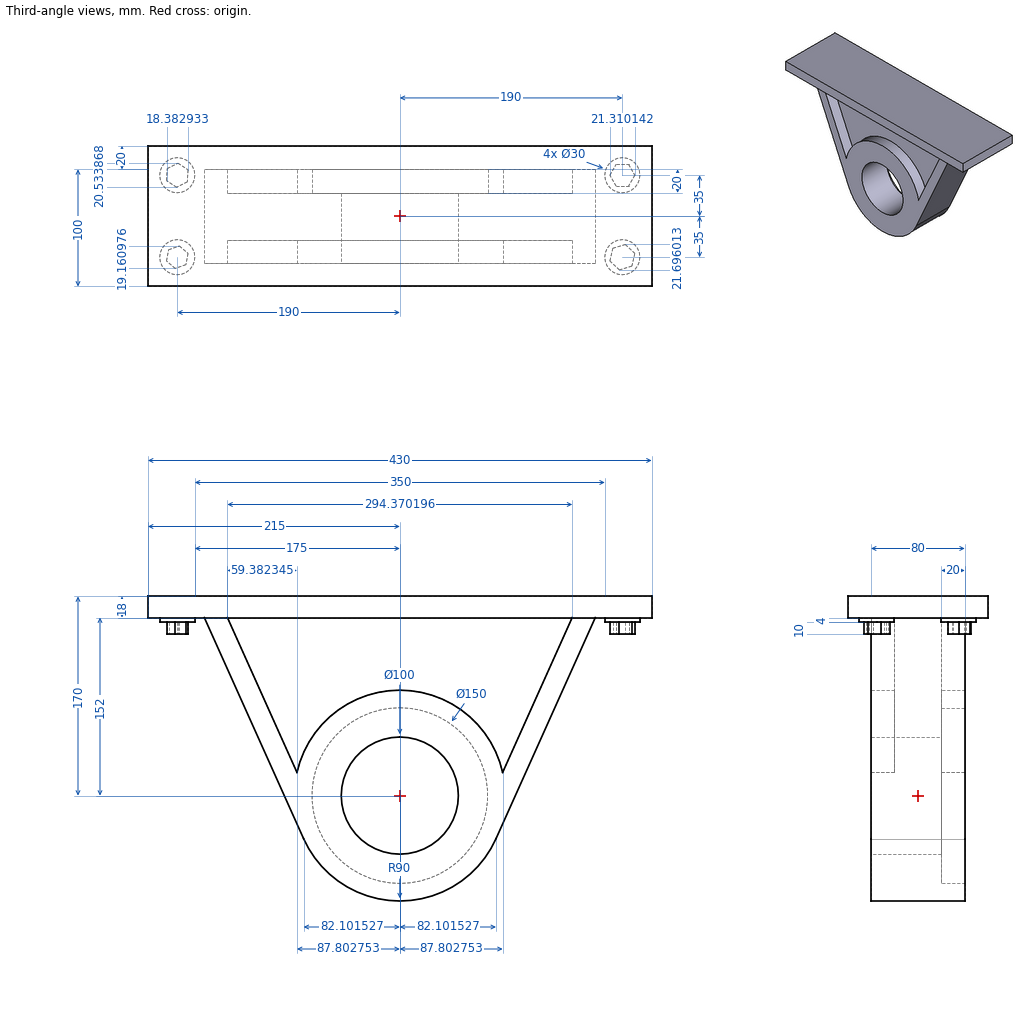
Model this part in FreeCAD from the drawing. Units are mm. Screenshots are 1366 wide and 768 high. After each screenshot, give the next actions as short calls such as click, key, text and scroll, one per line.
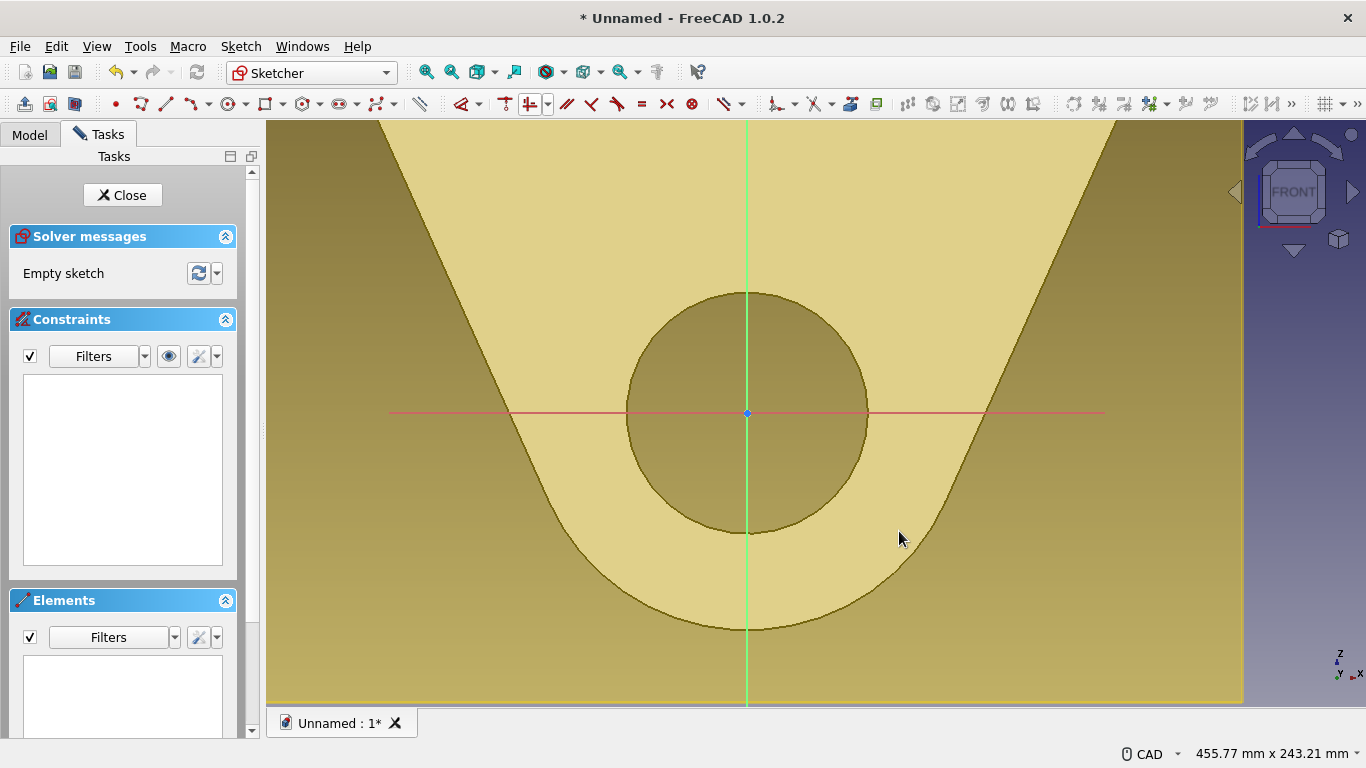
click(228, 104)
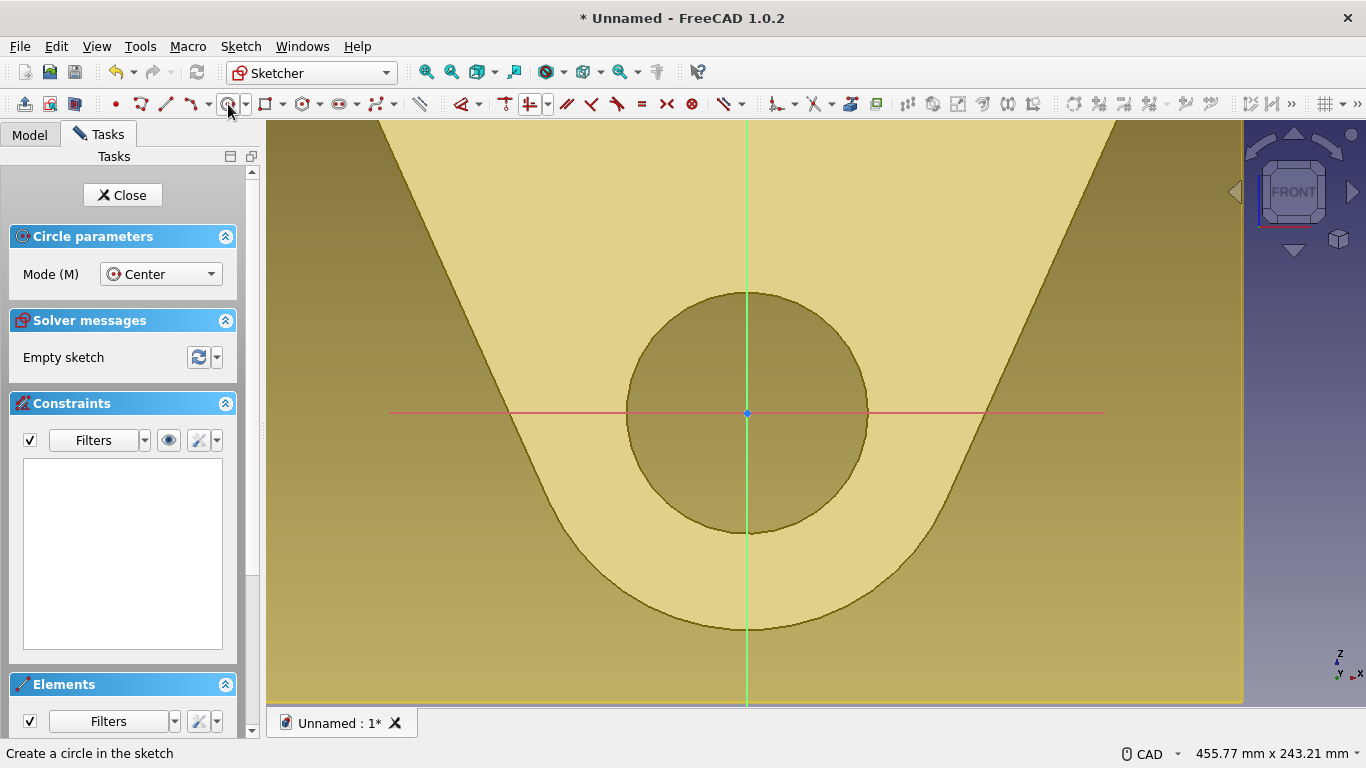
click(747, 413)
click(875, 285)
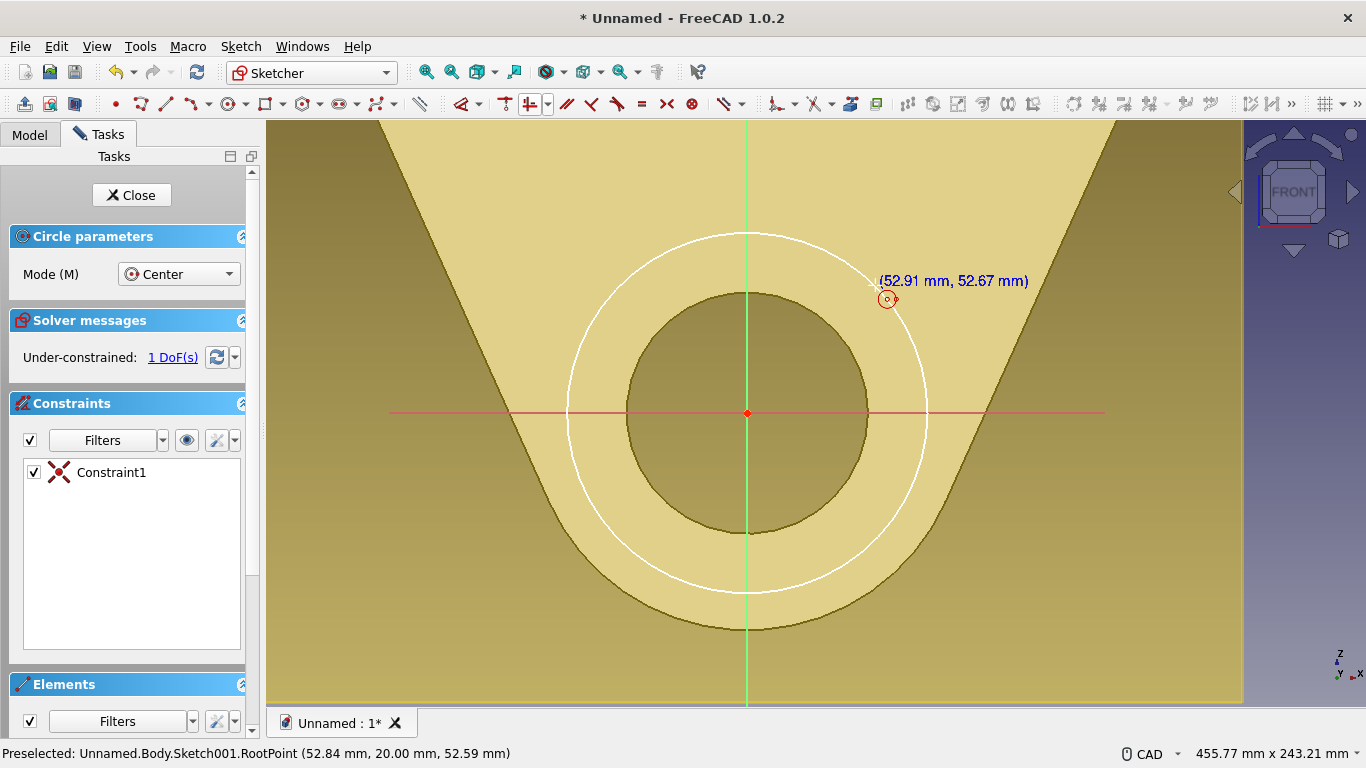
click(747, 413)
click(833, 328)
key(Escape)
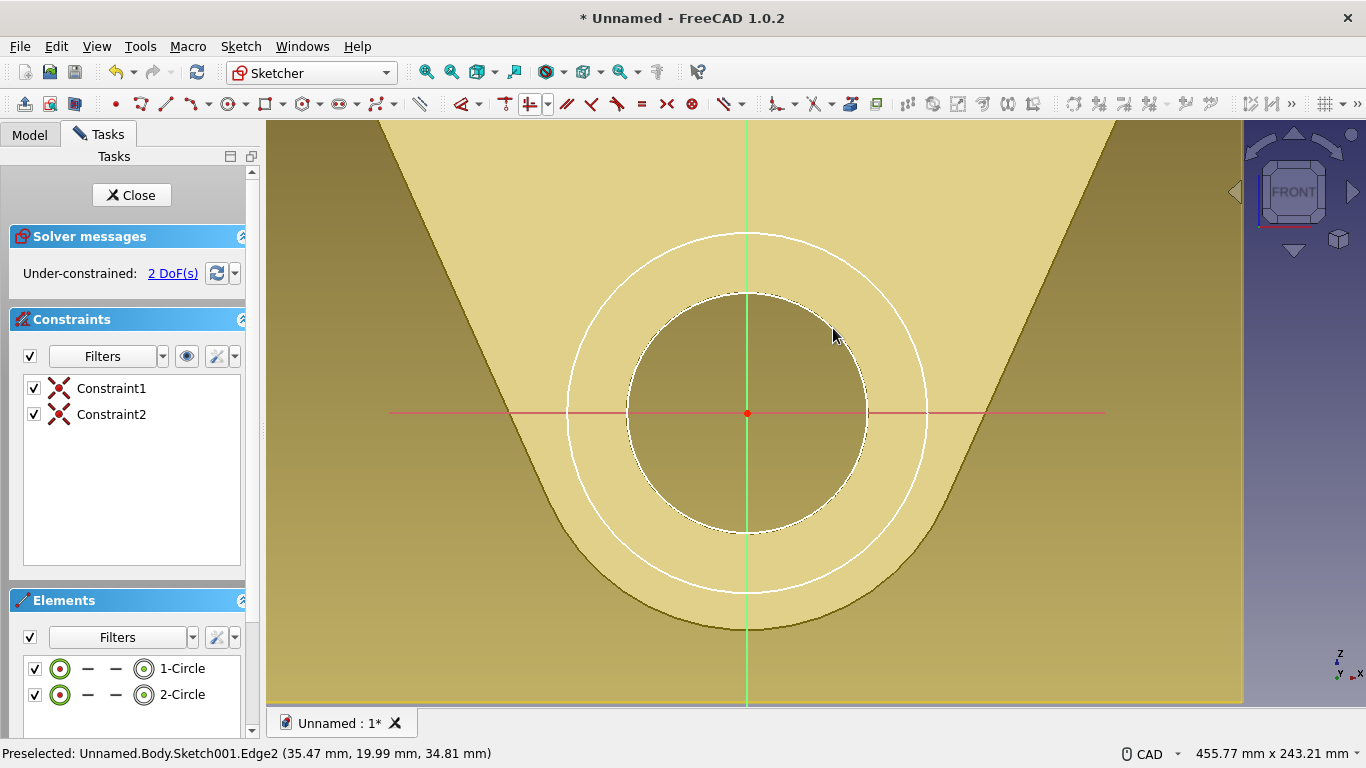
click(460, 104)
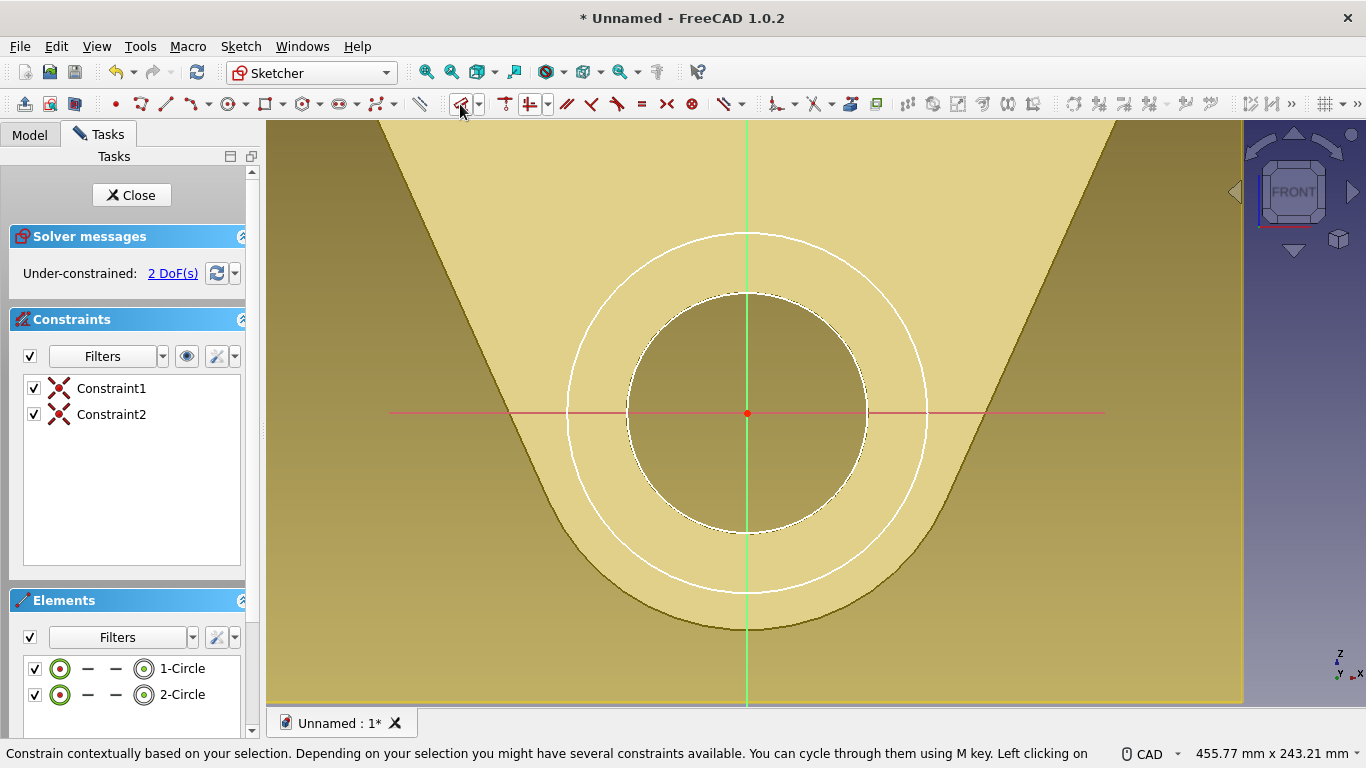
click(874, 285)
click(897, 262)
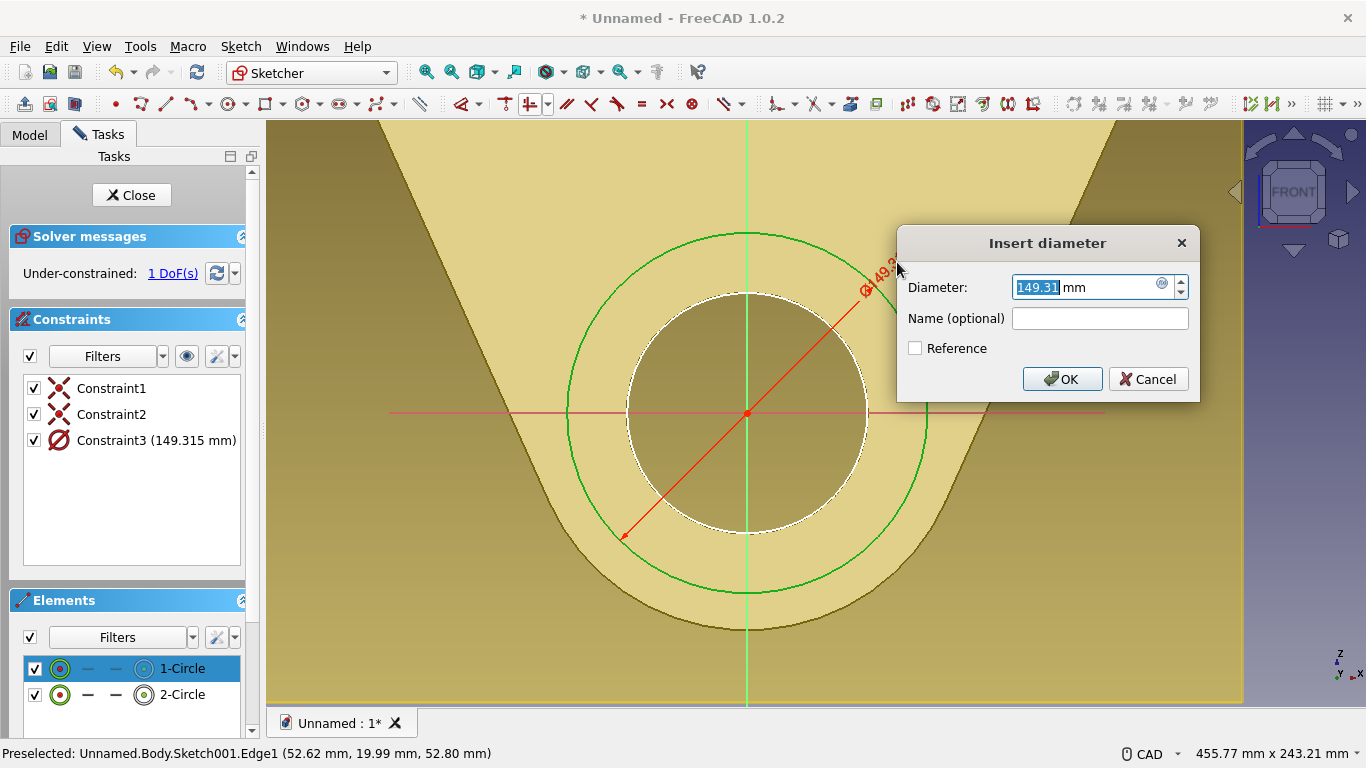
text(150)
key(Return)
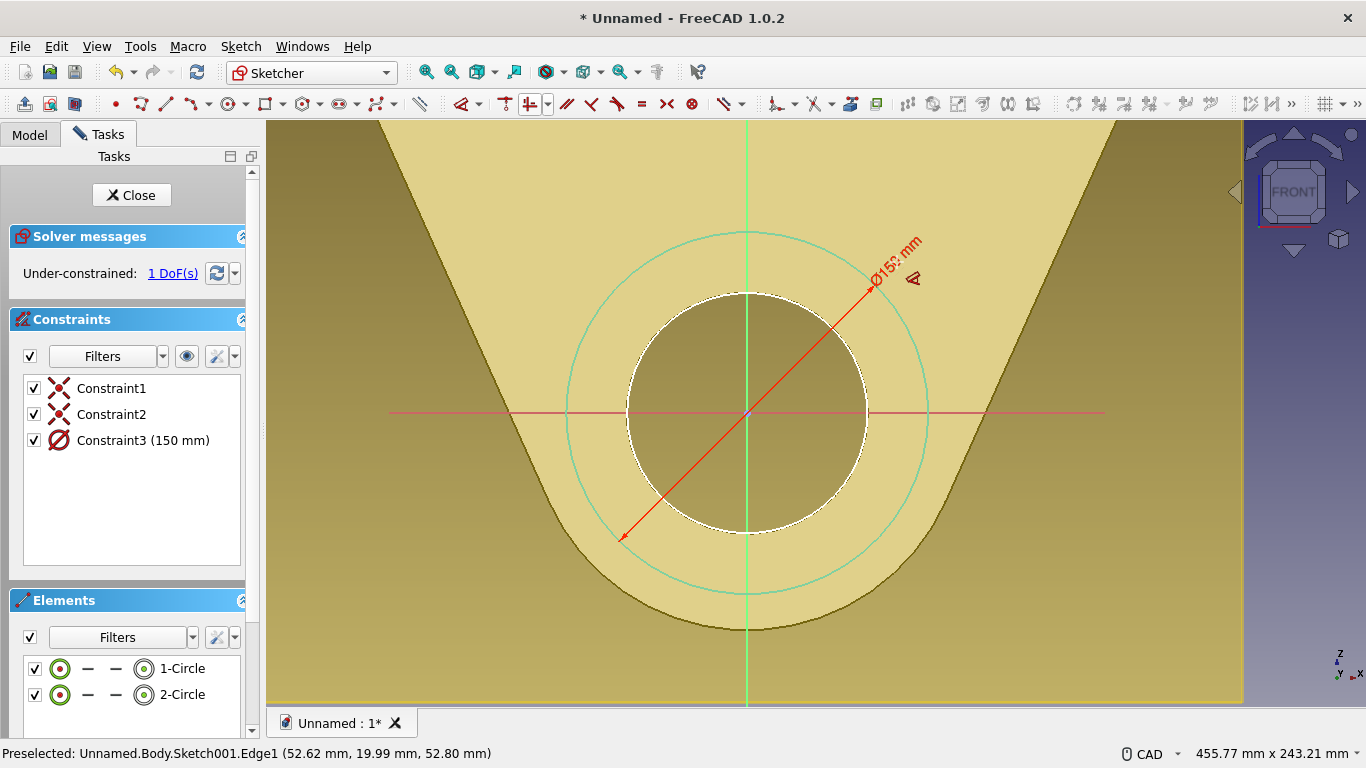
click(832, 328)
click(855, 305)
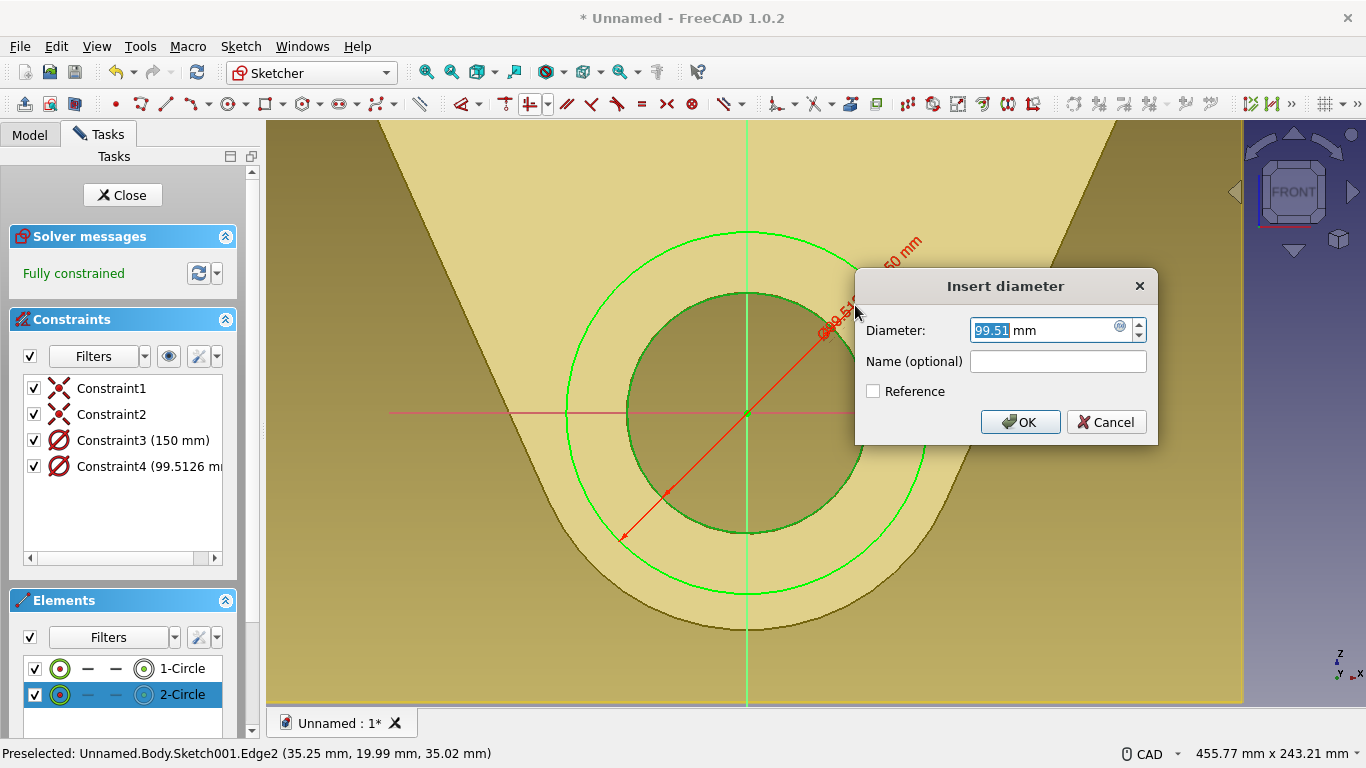
text(100)
key(Return)
key(Escape)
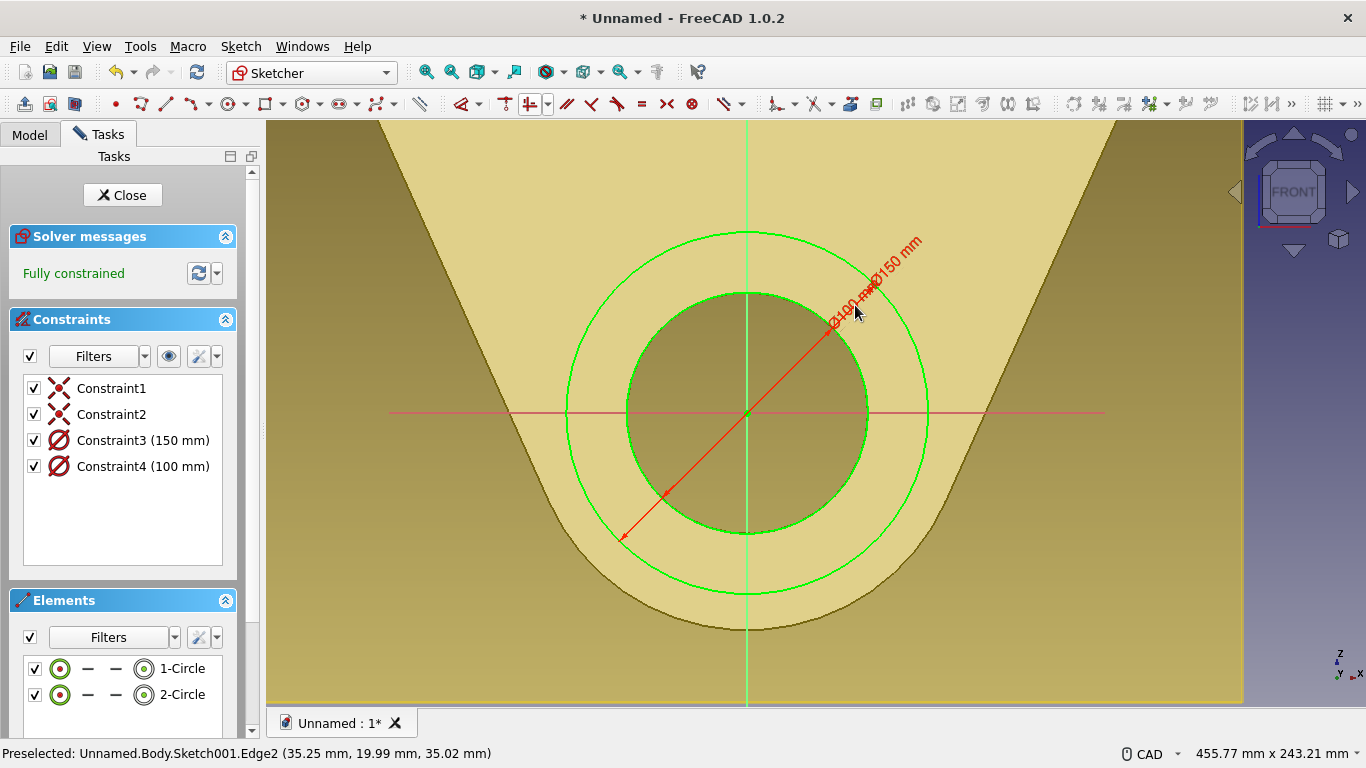
click(123, 195)